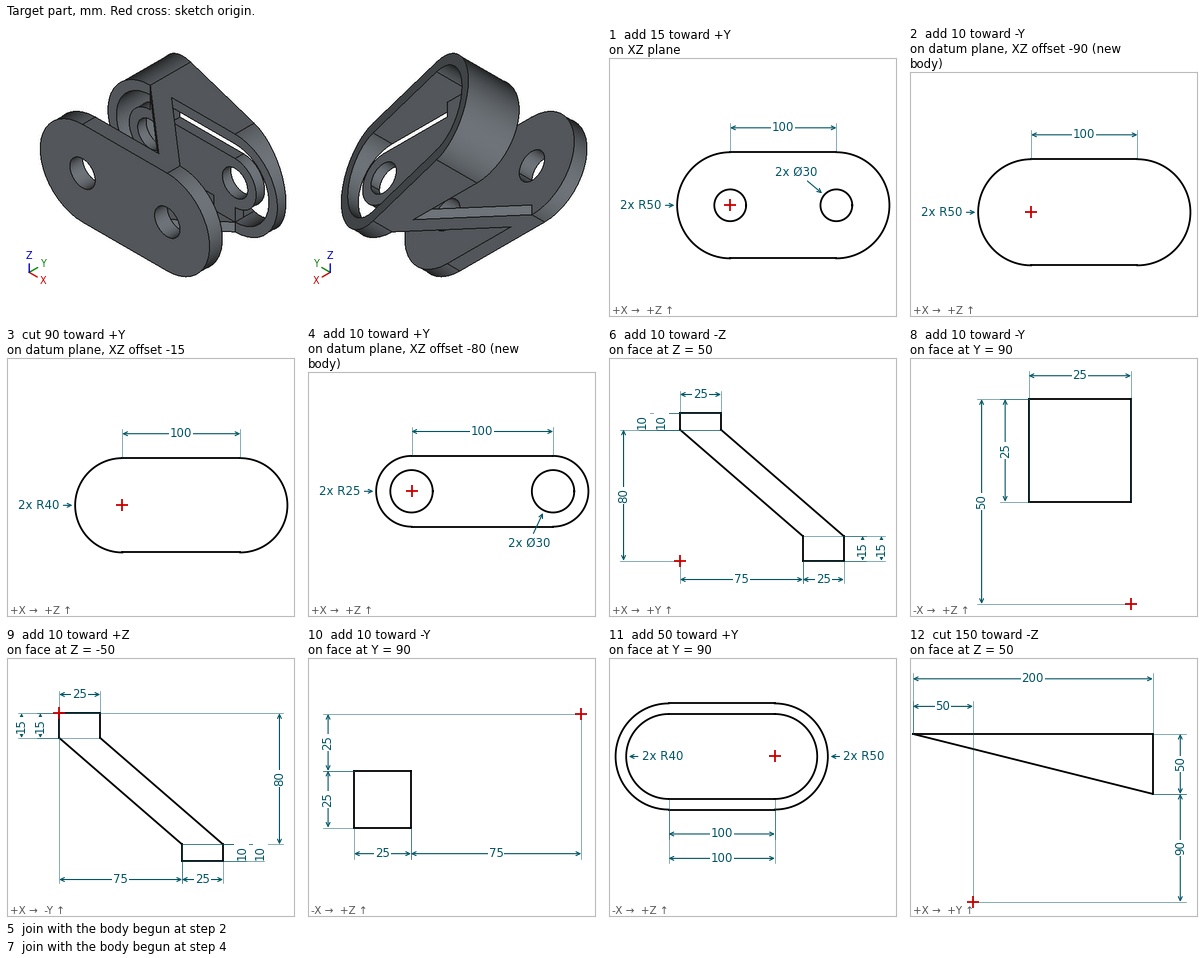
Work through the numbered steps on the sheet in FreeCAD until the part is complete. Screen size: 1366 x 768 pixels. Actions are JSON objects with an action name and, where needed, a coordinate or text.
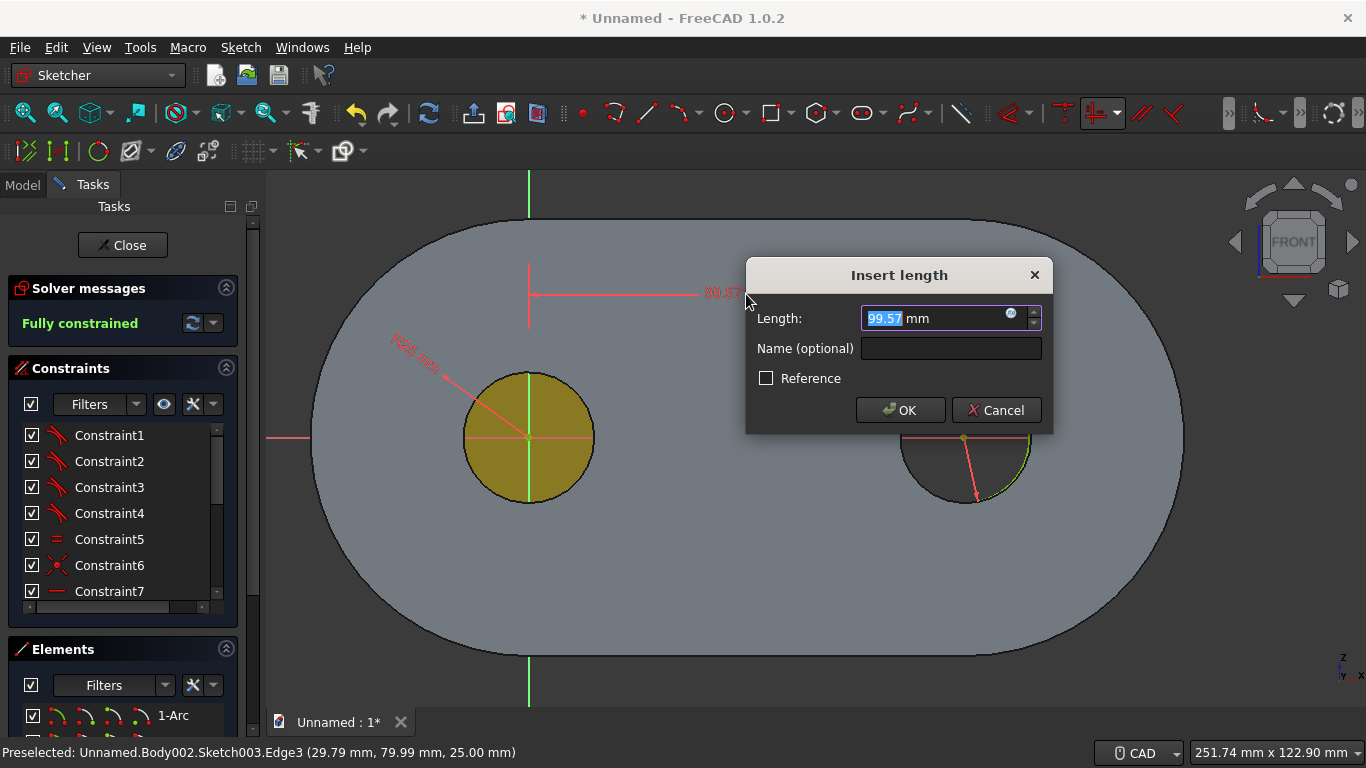
{"action": "type", "text": "100"}
{"action": "key", "text": "Return"}
{"action": "key", "text": "Escape"}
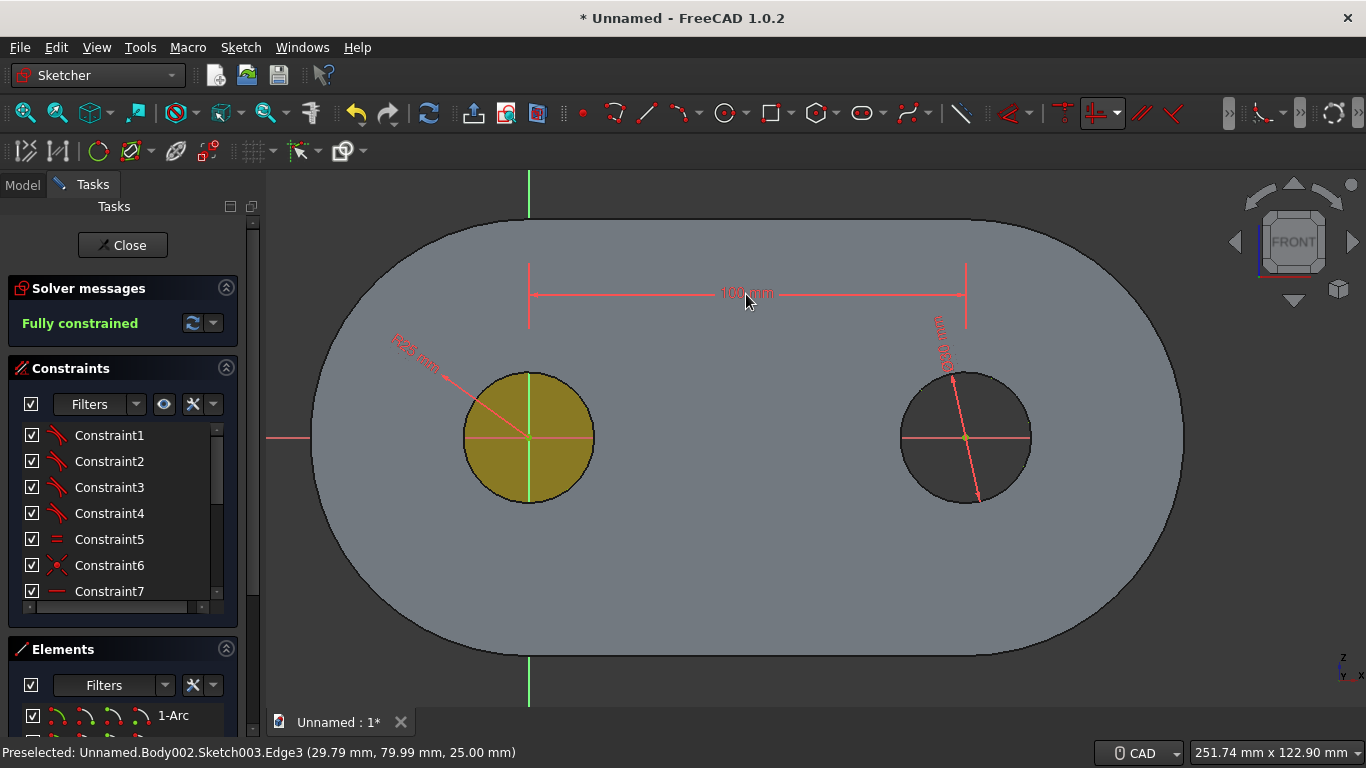
{"action": "left_click", "coordinate": [123, 245]}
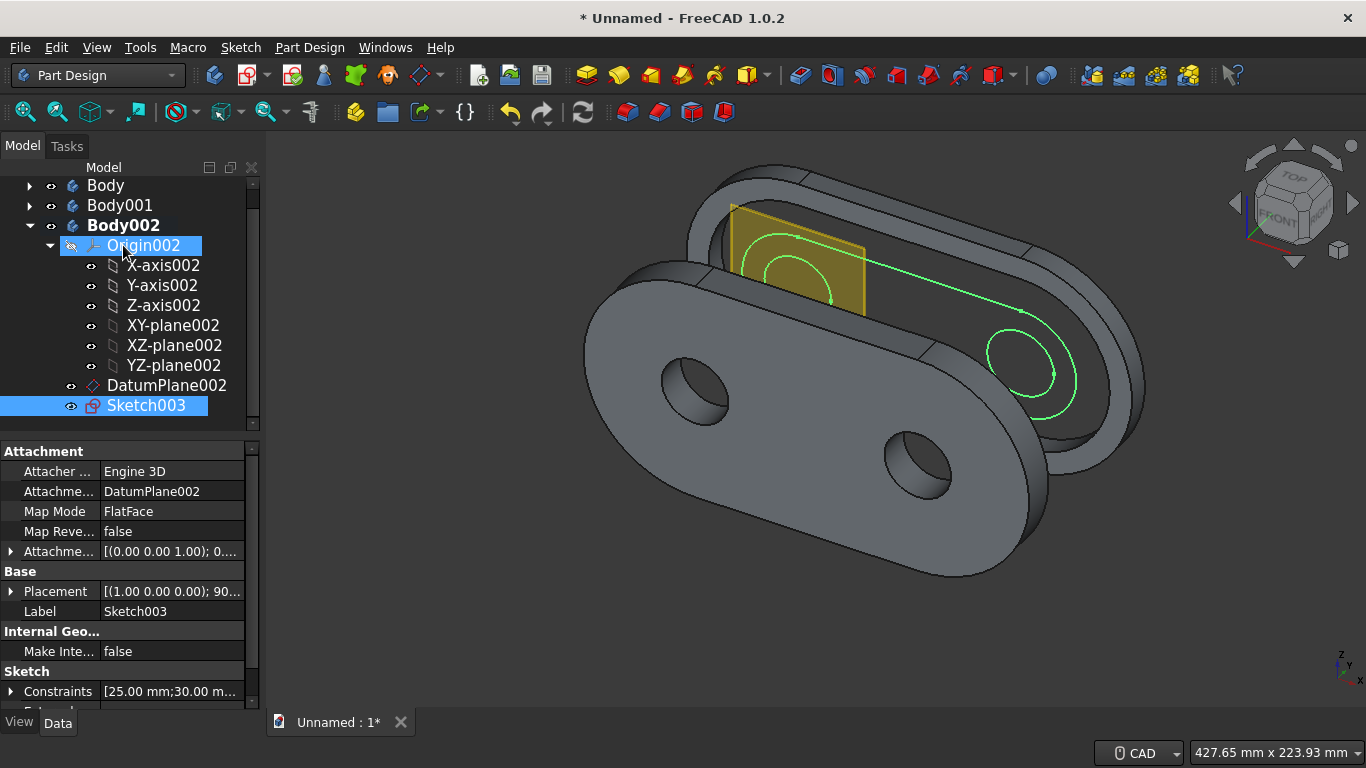
{"action": "left_click", "coordinate": [588, 76]}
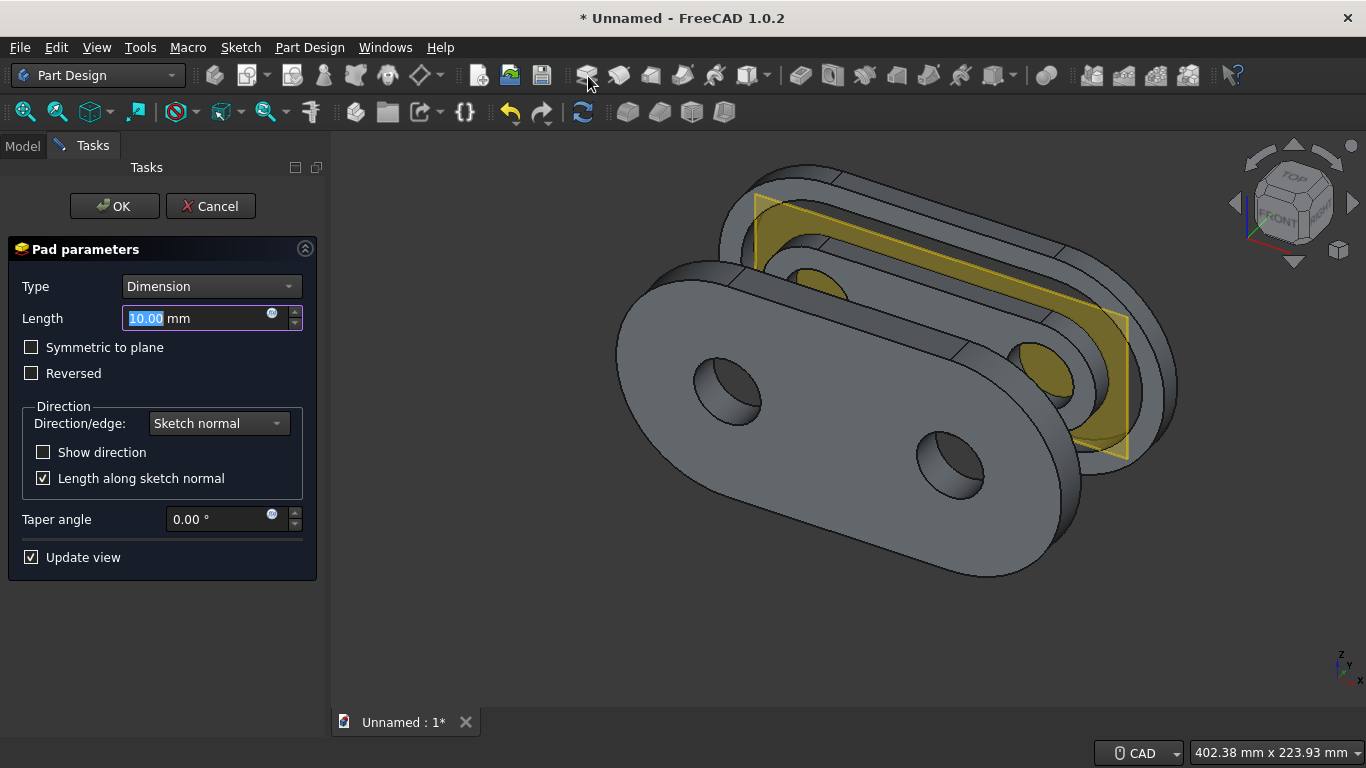
{"action": "type", "text": "10"}
{"action": "key", "text": "Tab"}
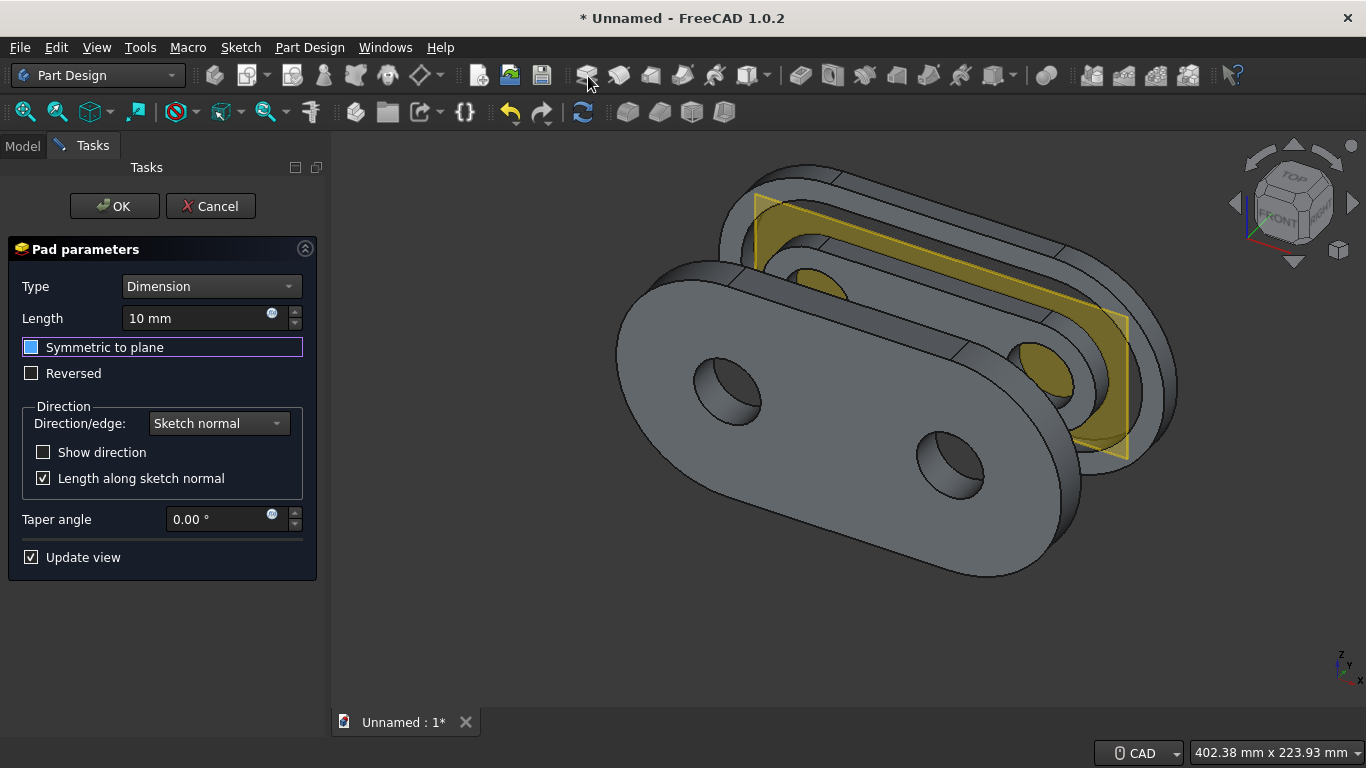
{"action": "left_click", "coordinate": [30, 373]}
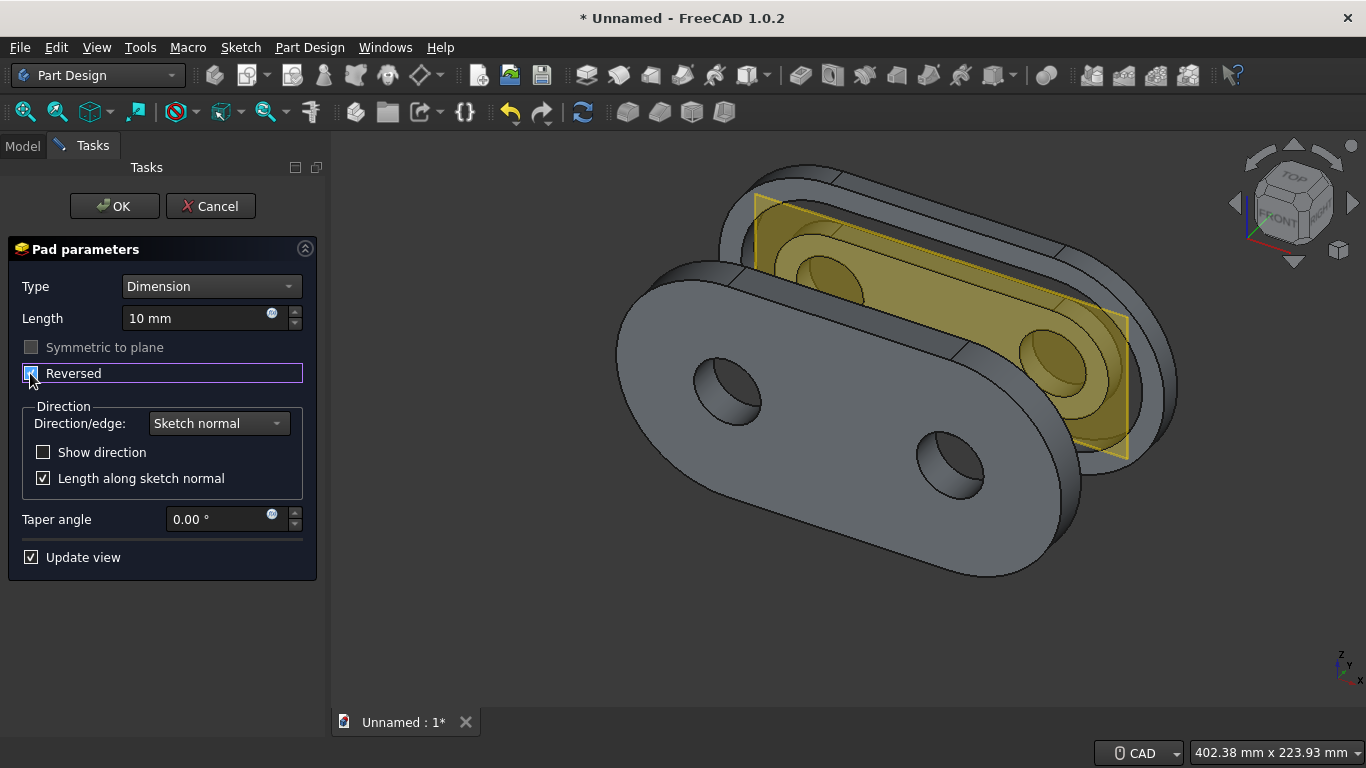
{"action": "left_click", "coordinate": [115, 206]}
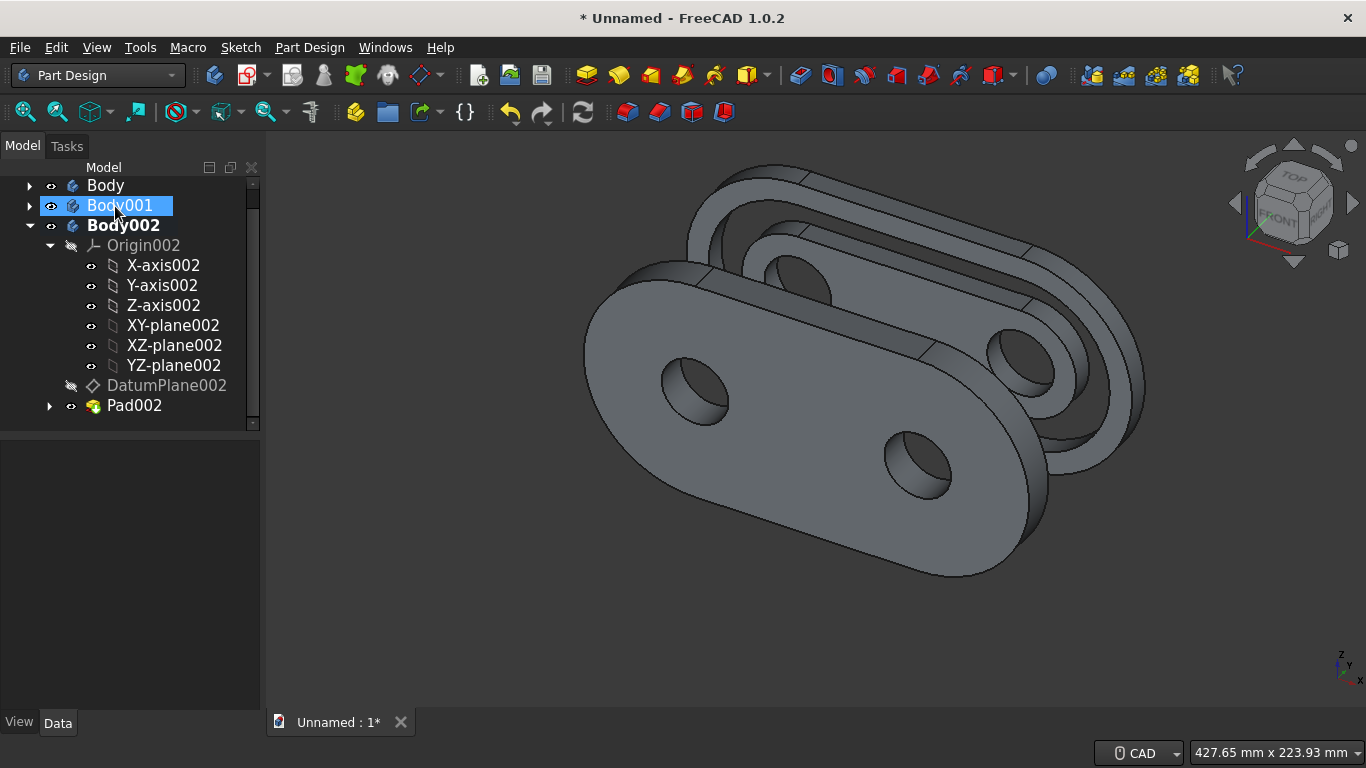
{"action": "left_click", "coordinate": [26, 112]}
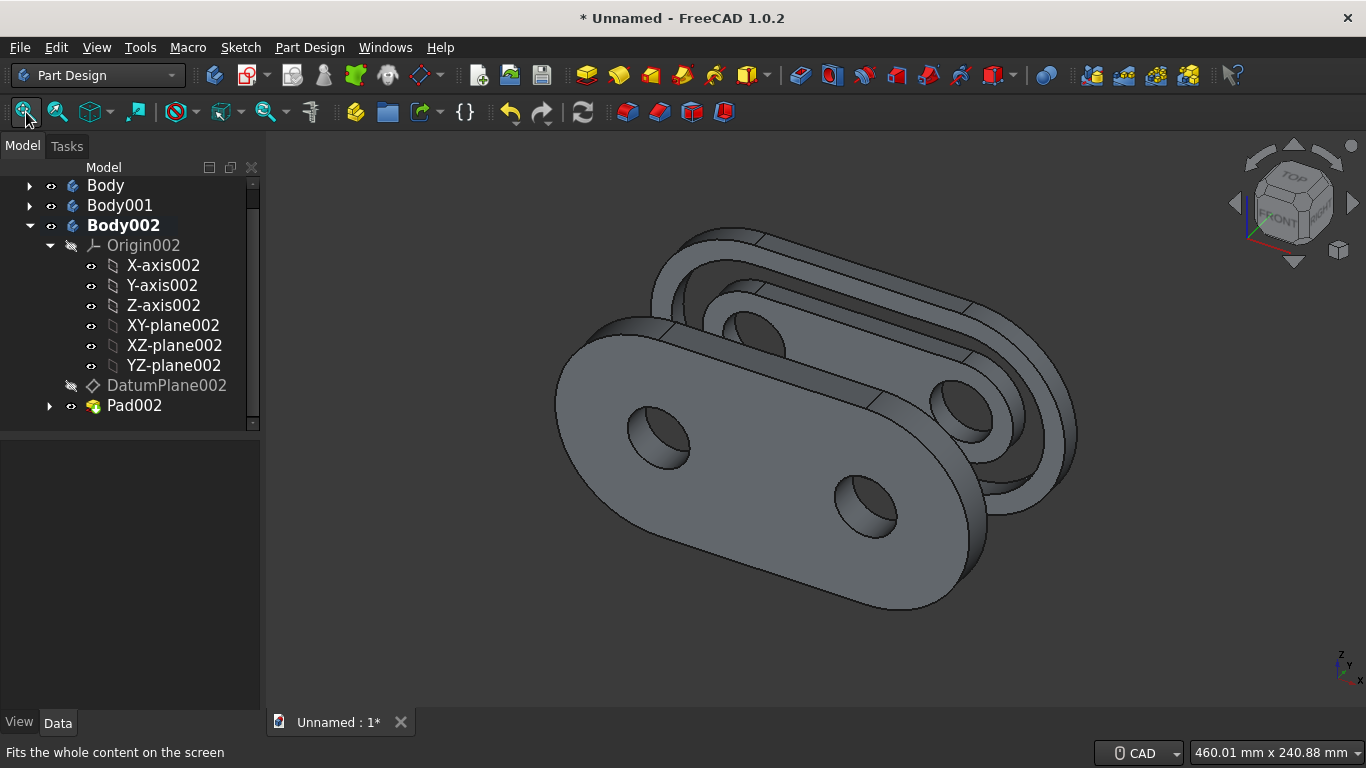
{"action": "double_click", "coordinate": [96, 186]}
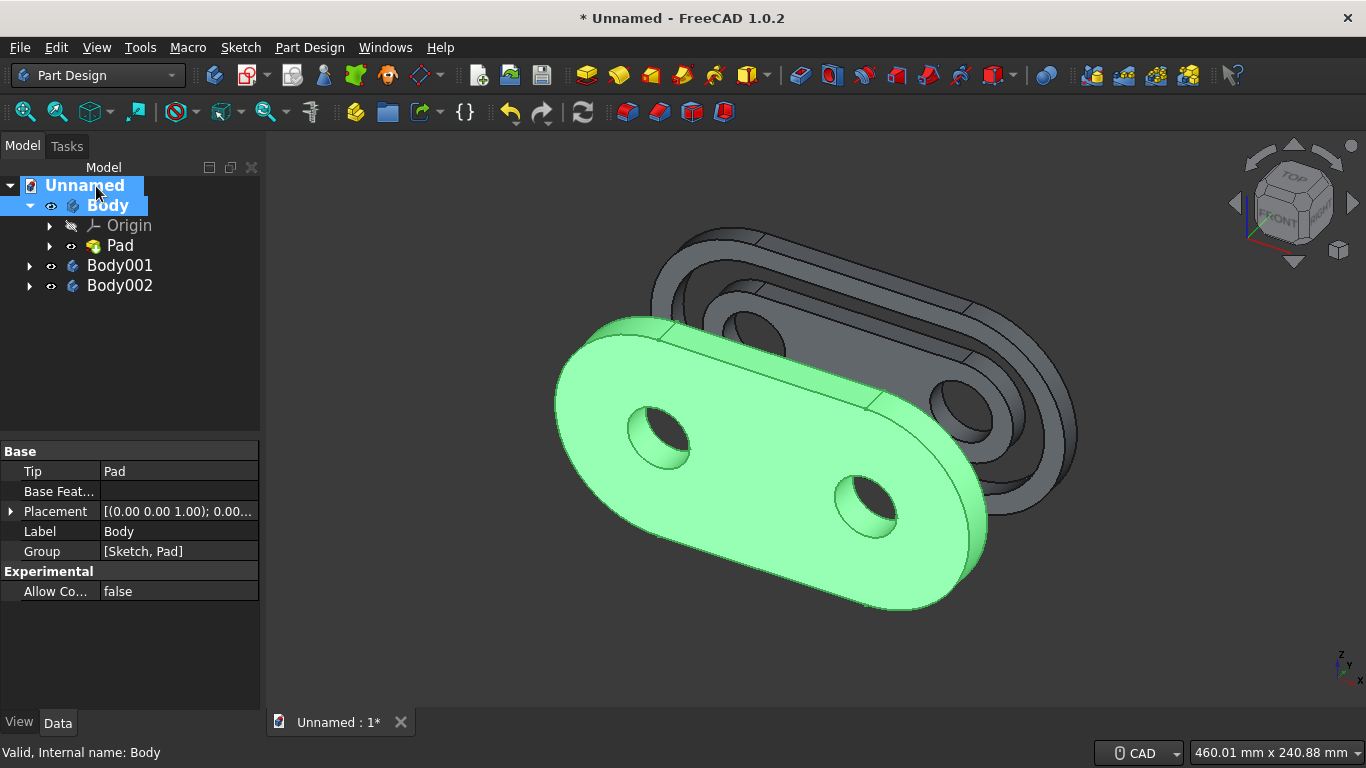
{"action": "left_click", "coordinate": [96, 206]}